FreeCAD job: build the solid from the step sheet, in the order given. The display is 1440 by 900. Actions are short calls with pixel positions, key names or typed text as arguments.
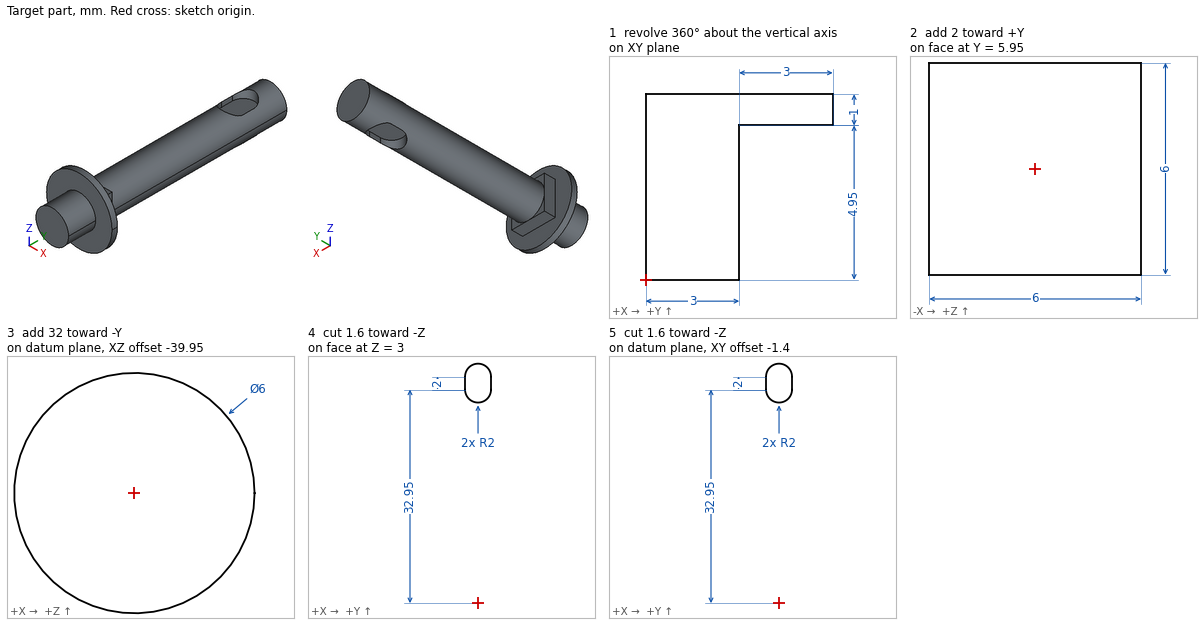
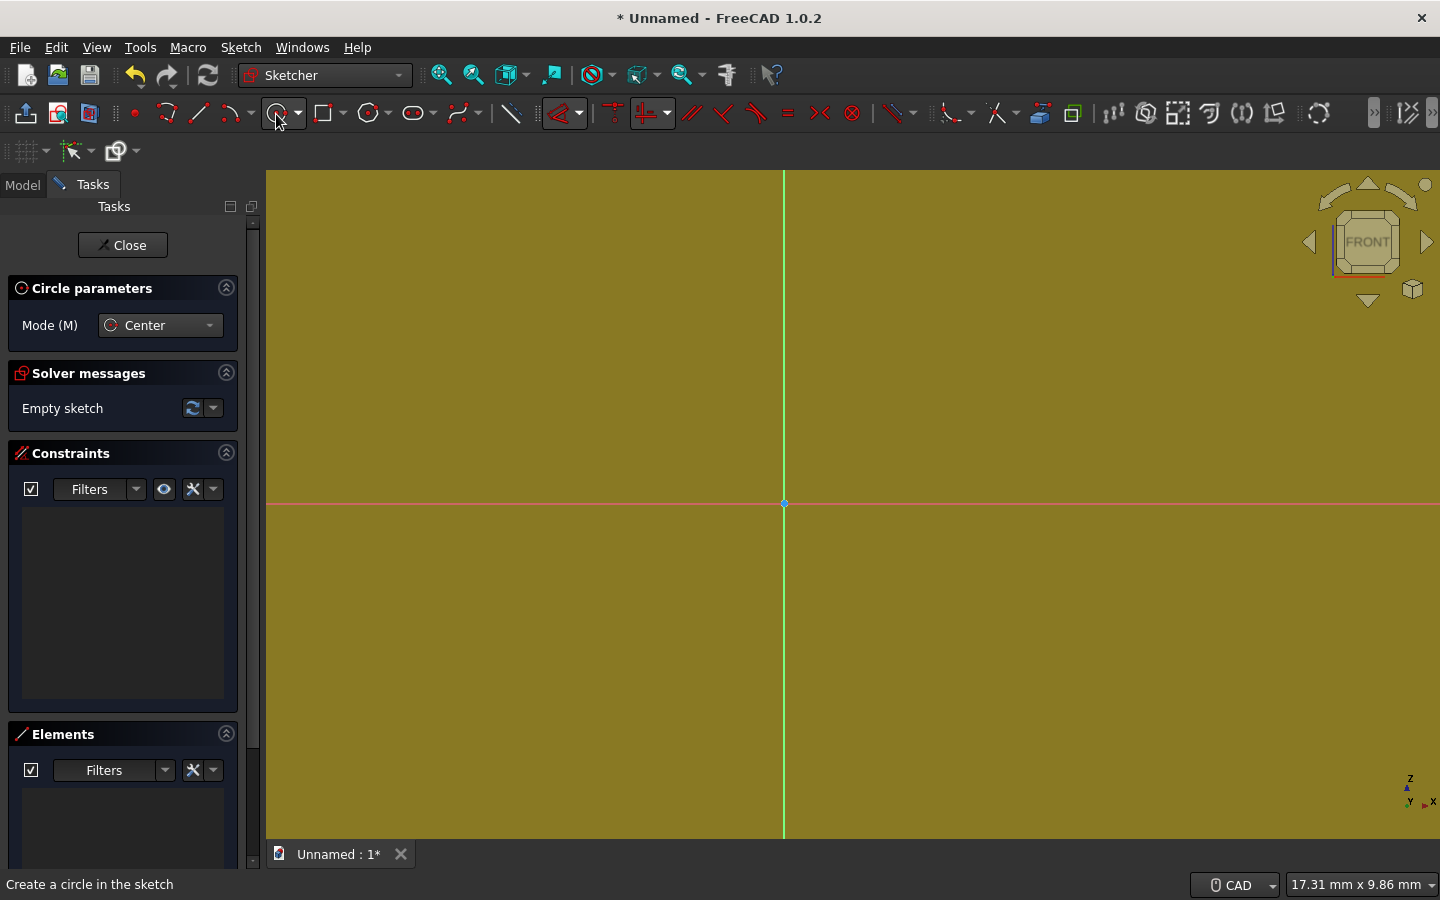
click(784, 504)
click(928, 360)
key(Escape)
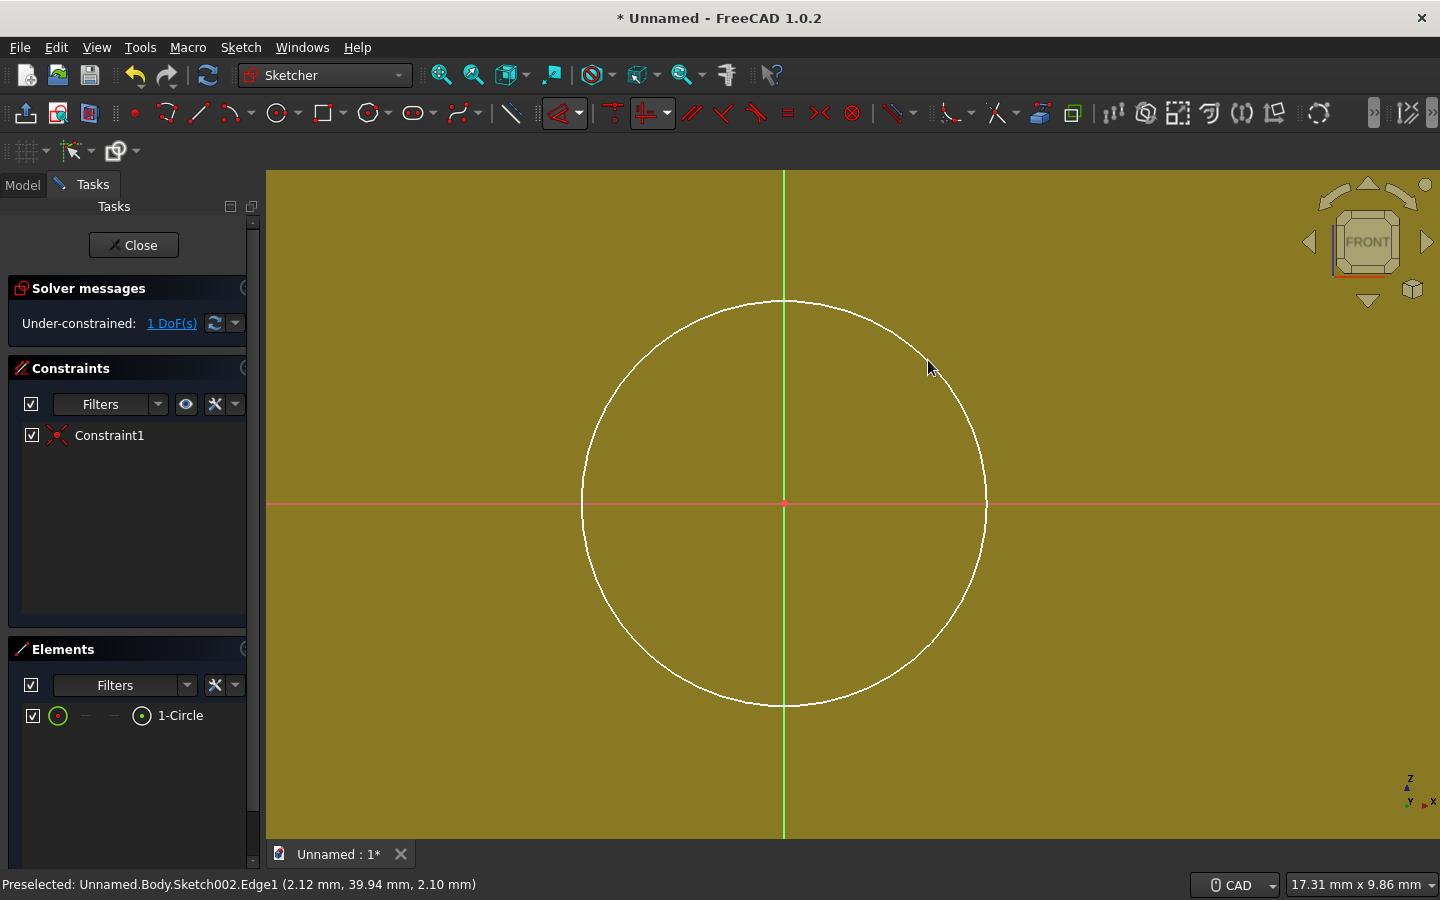
click(927, 360)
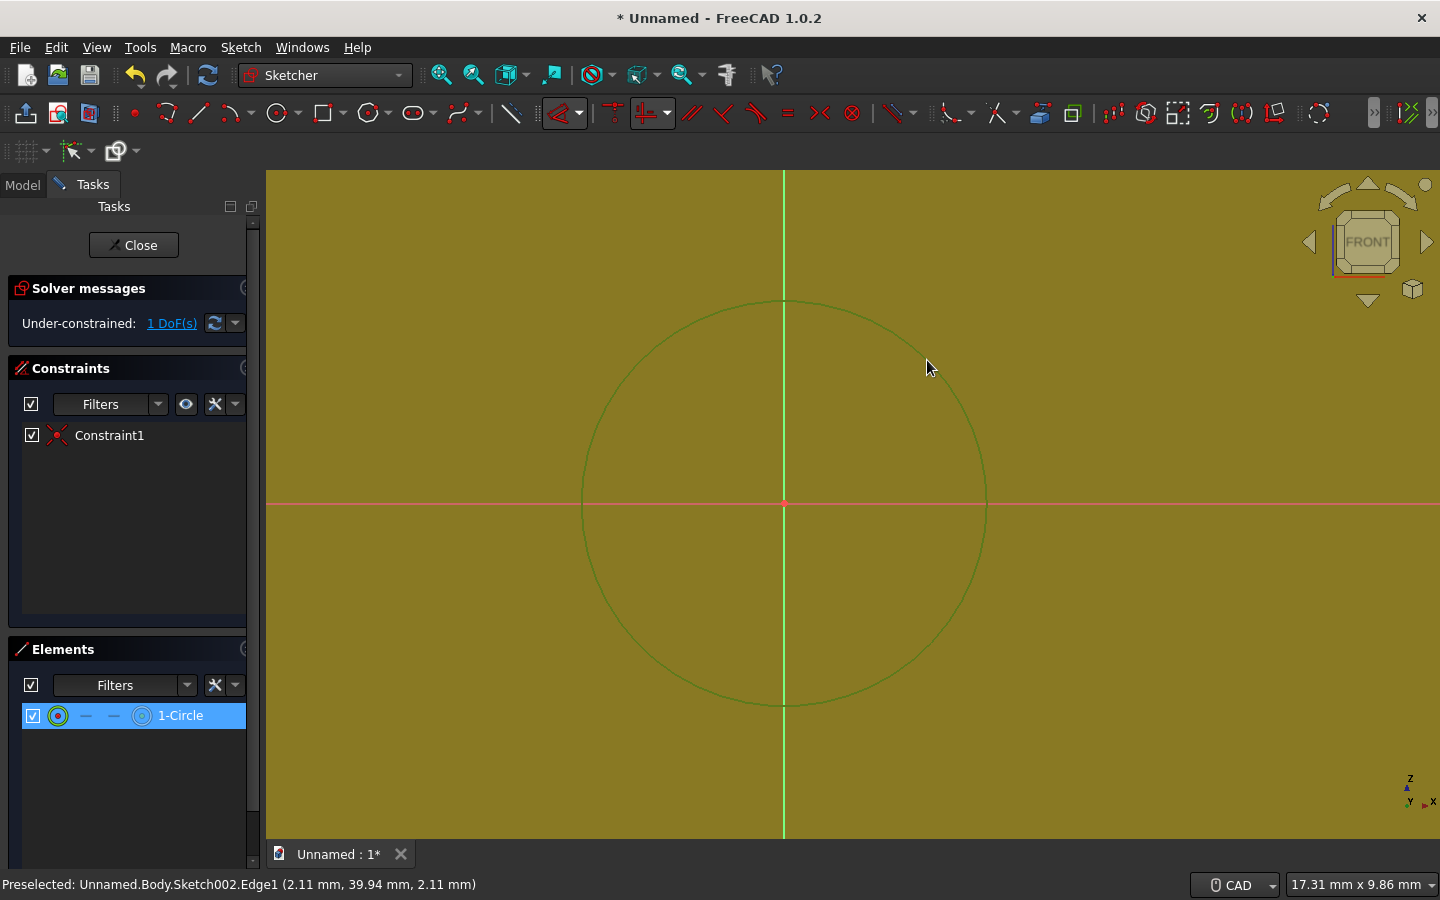
key(k)
key(o)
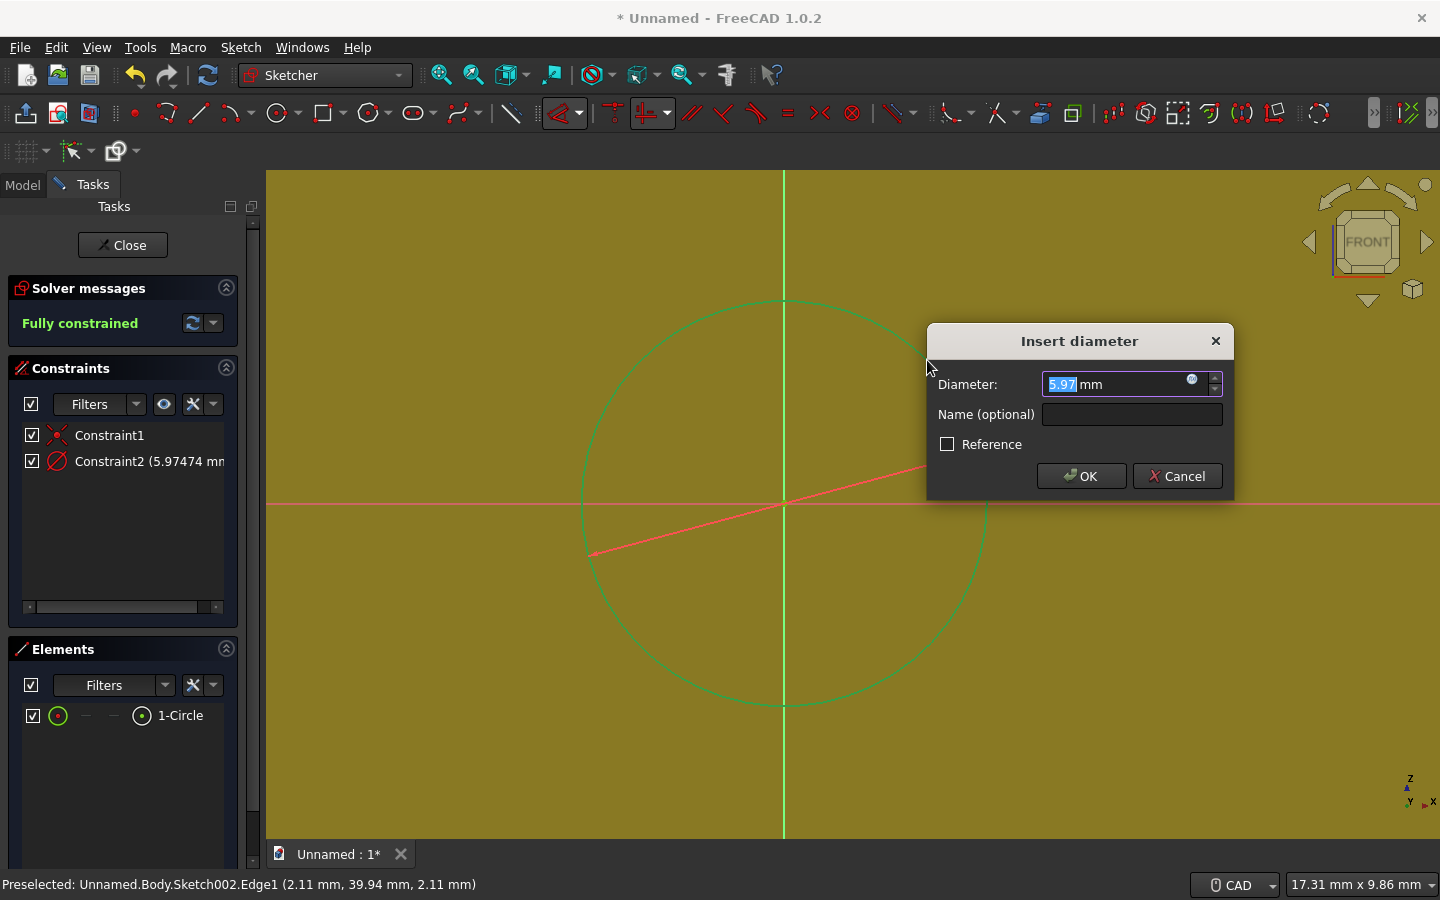
text(6)
key(Return)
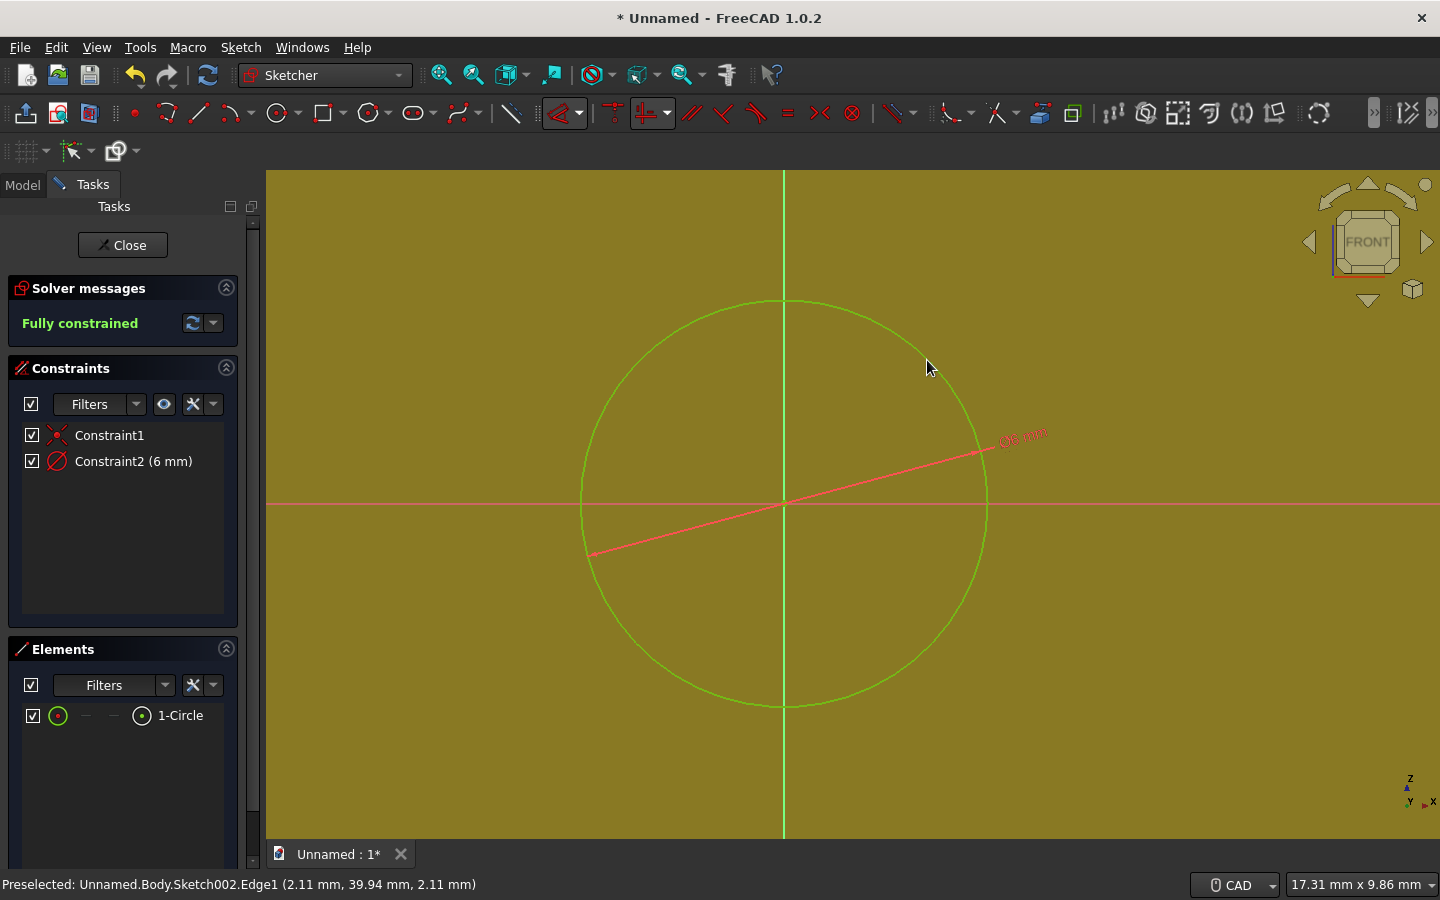
click(123, 245)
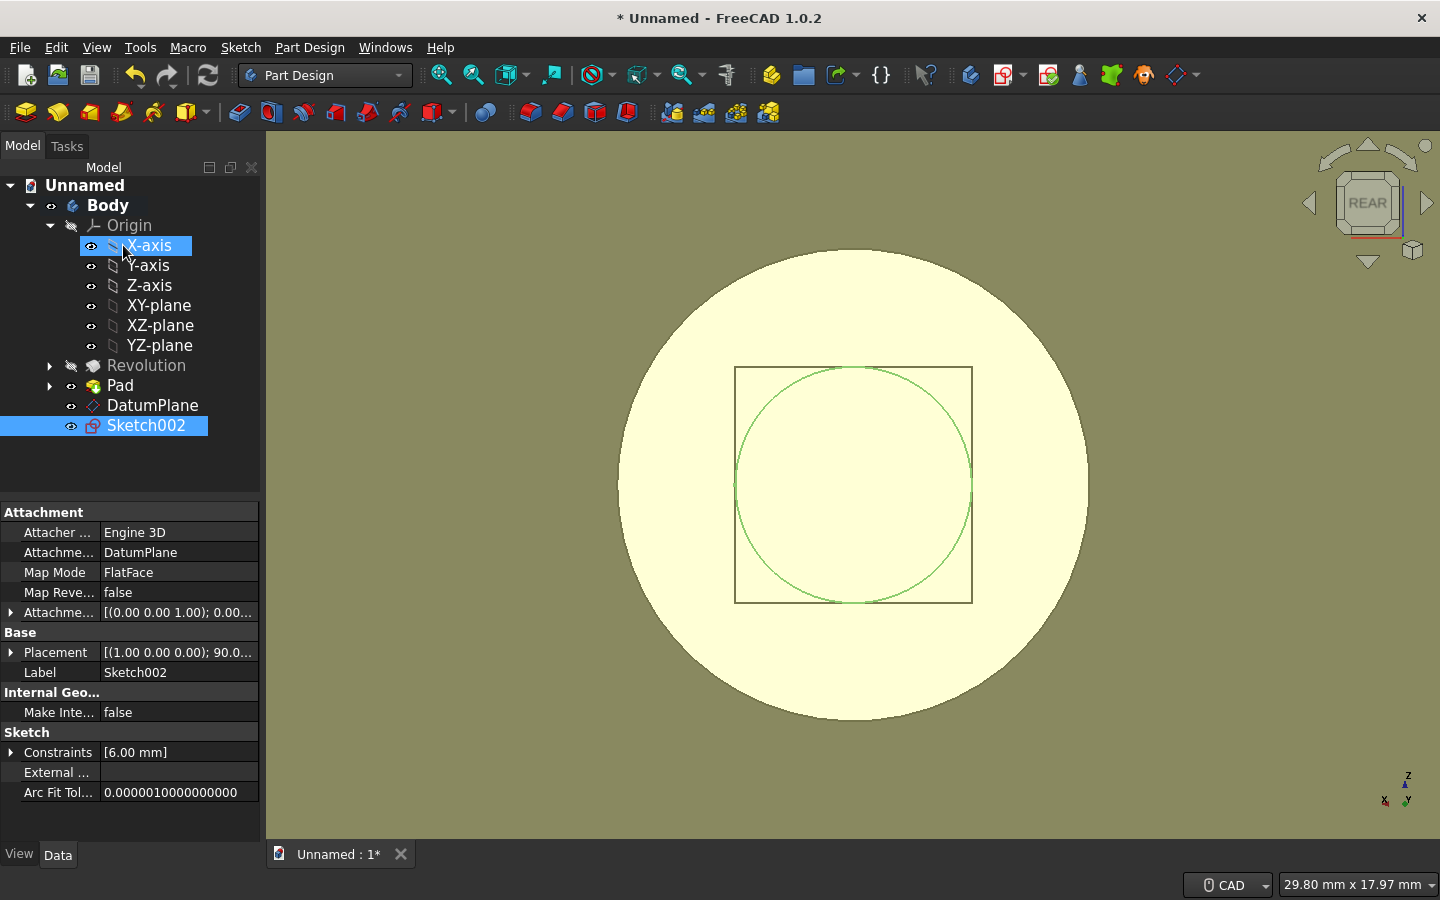
click(26, 112)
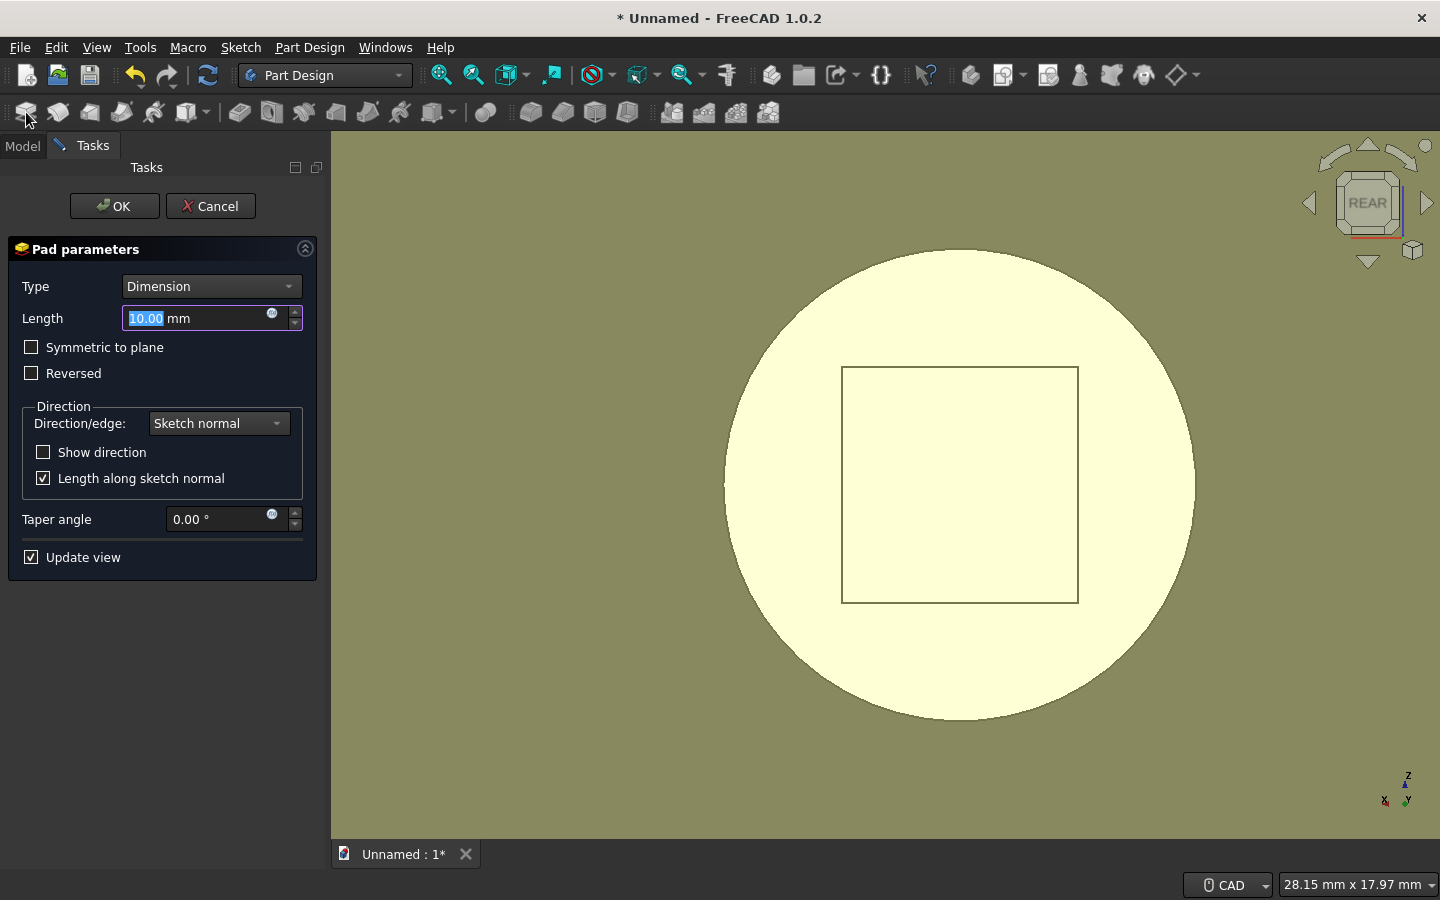
text(32)
key(Tab)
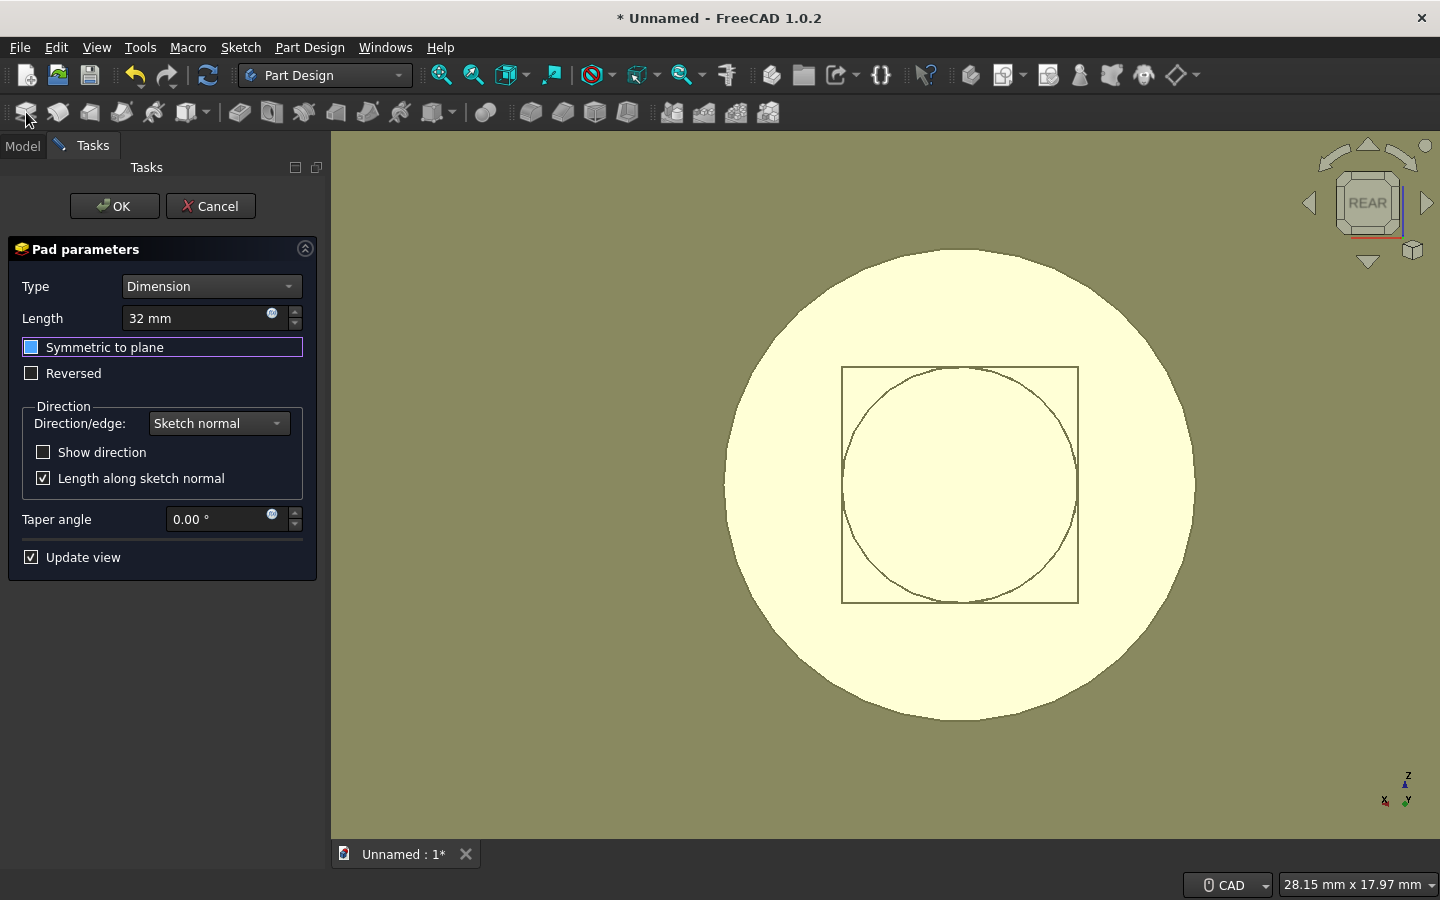
click(115, 206)